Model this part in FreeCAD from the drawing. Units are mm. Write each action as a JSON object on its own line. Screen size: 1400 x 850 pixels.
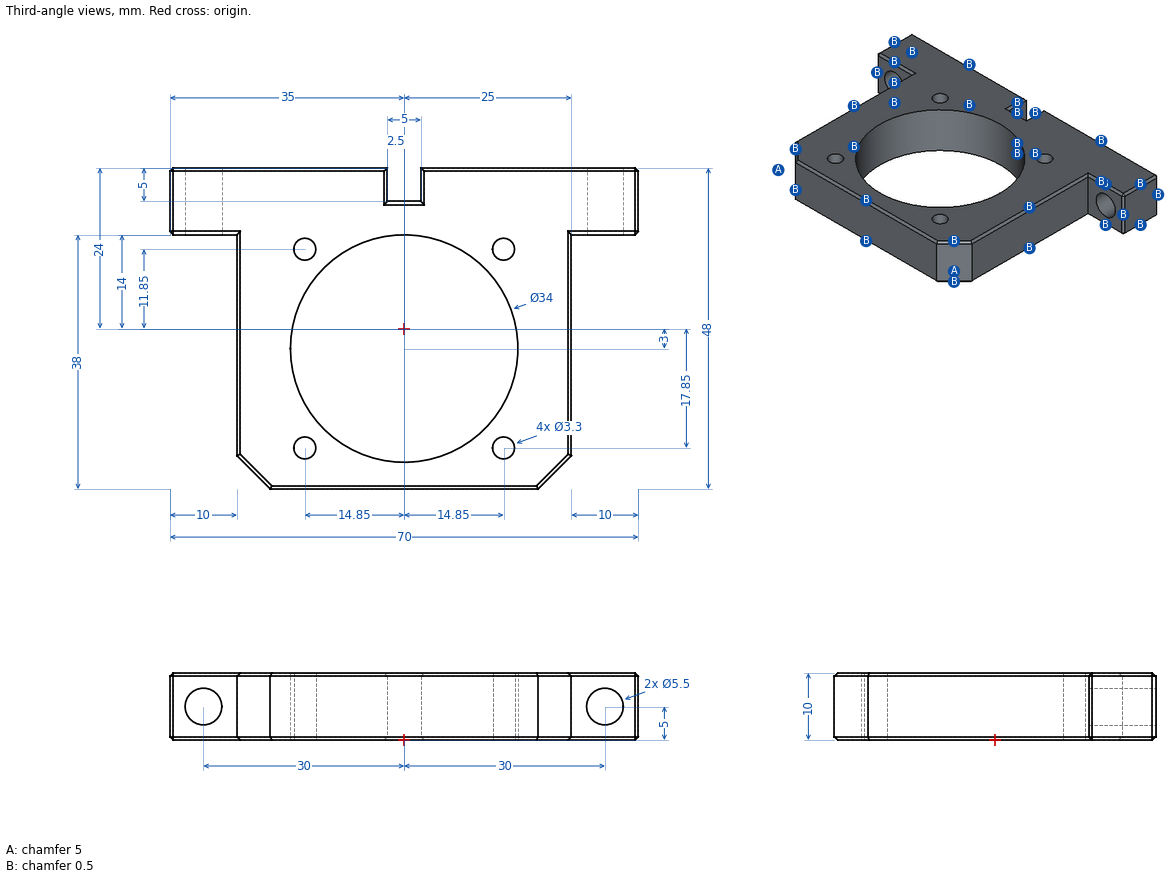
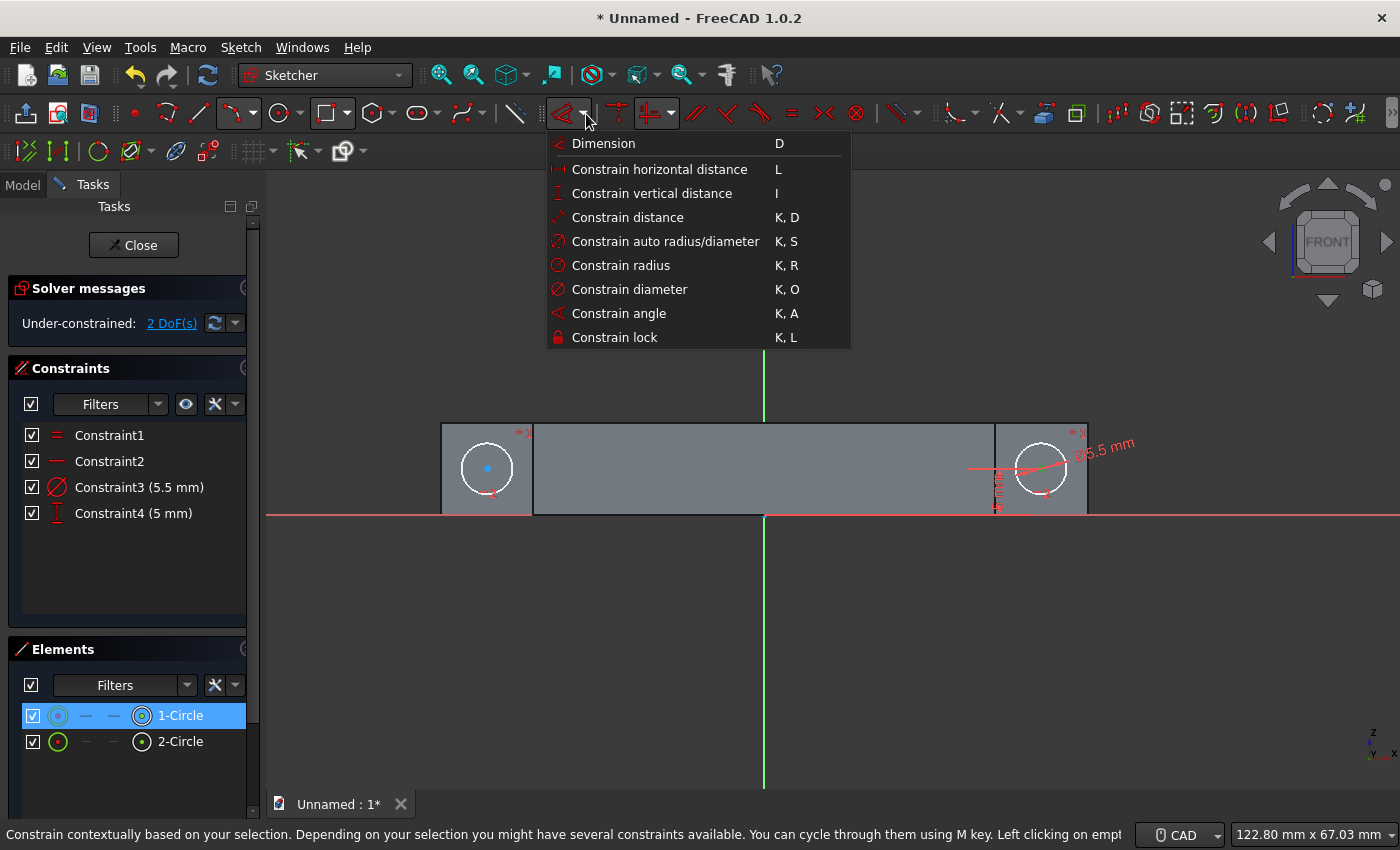
{"action": "left_click", "coordinate": [699, 169]}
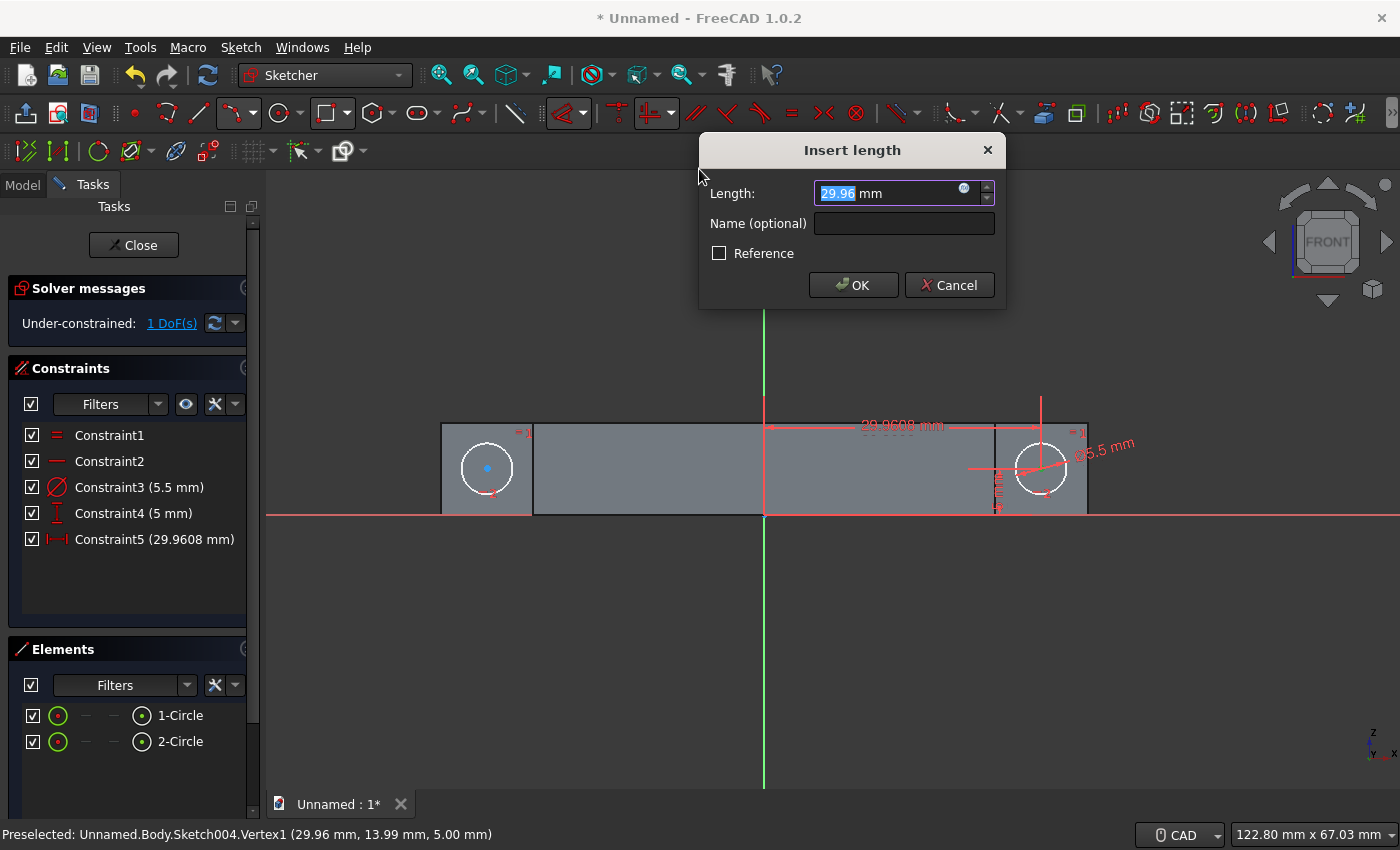
{"action": "type", "text": "30"}
{"action": "key", "text": "Return"}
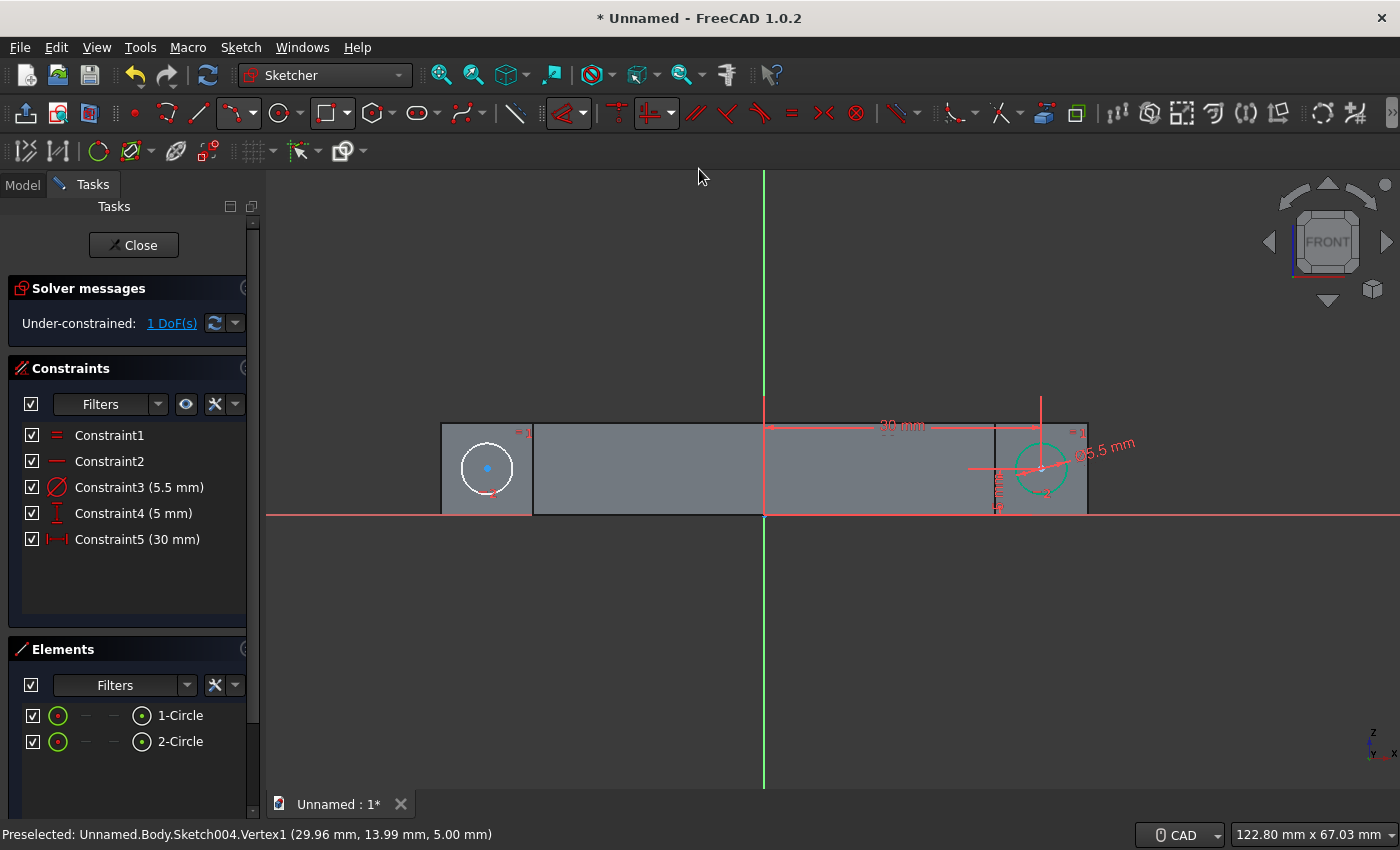
{"action": "left_click", "coordinate": [487, 469]}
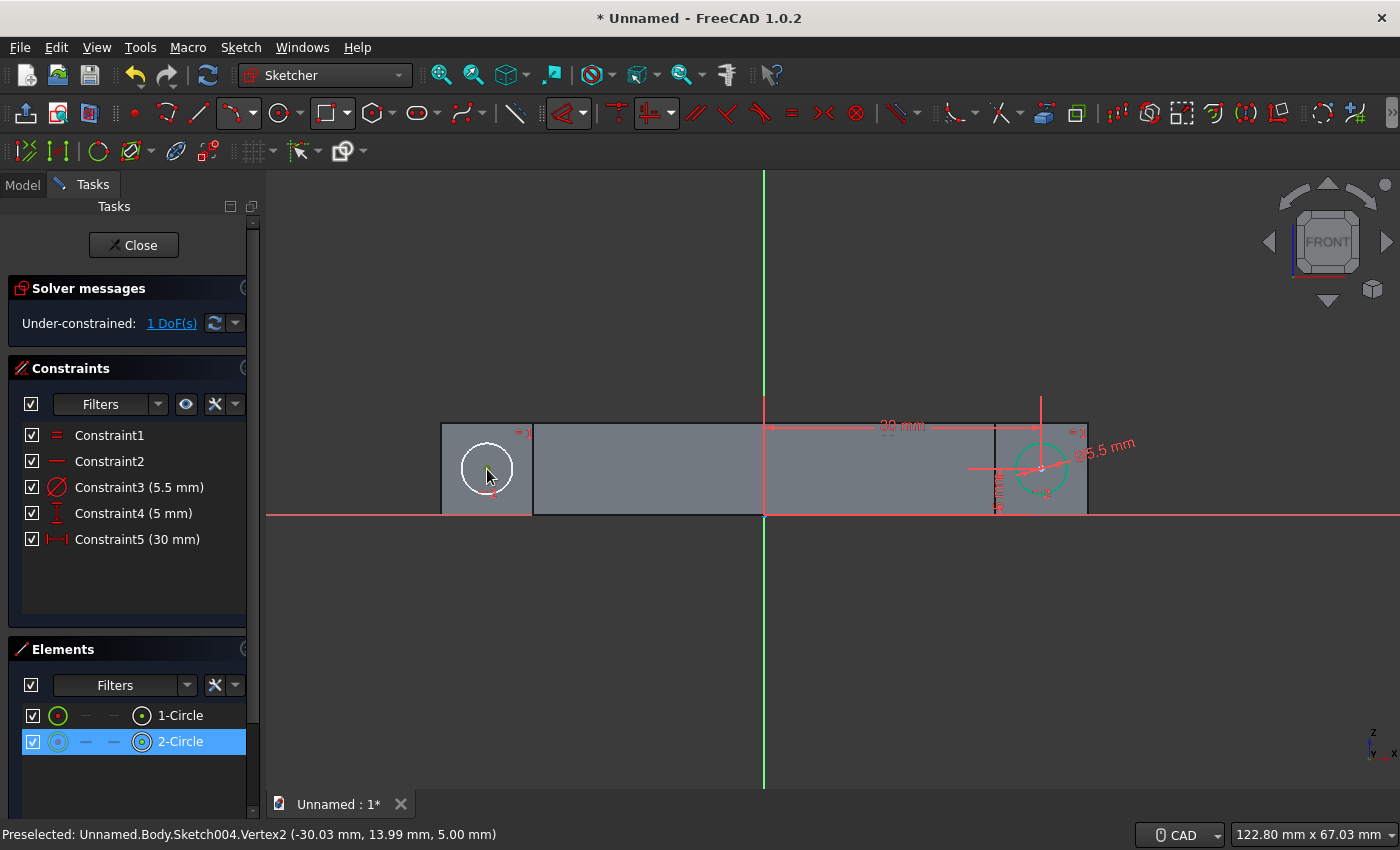
{"action": "key", "text": "l"}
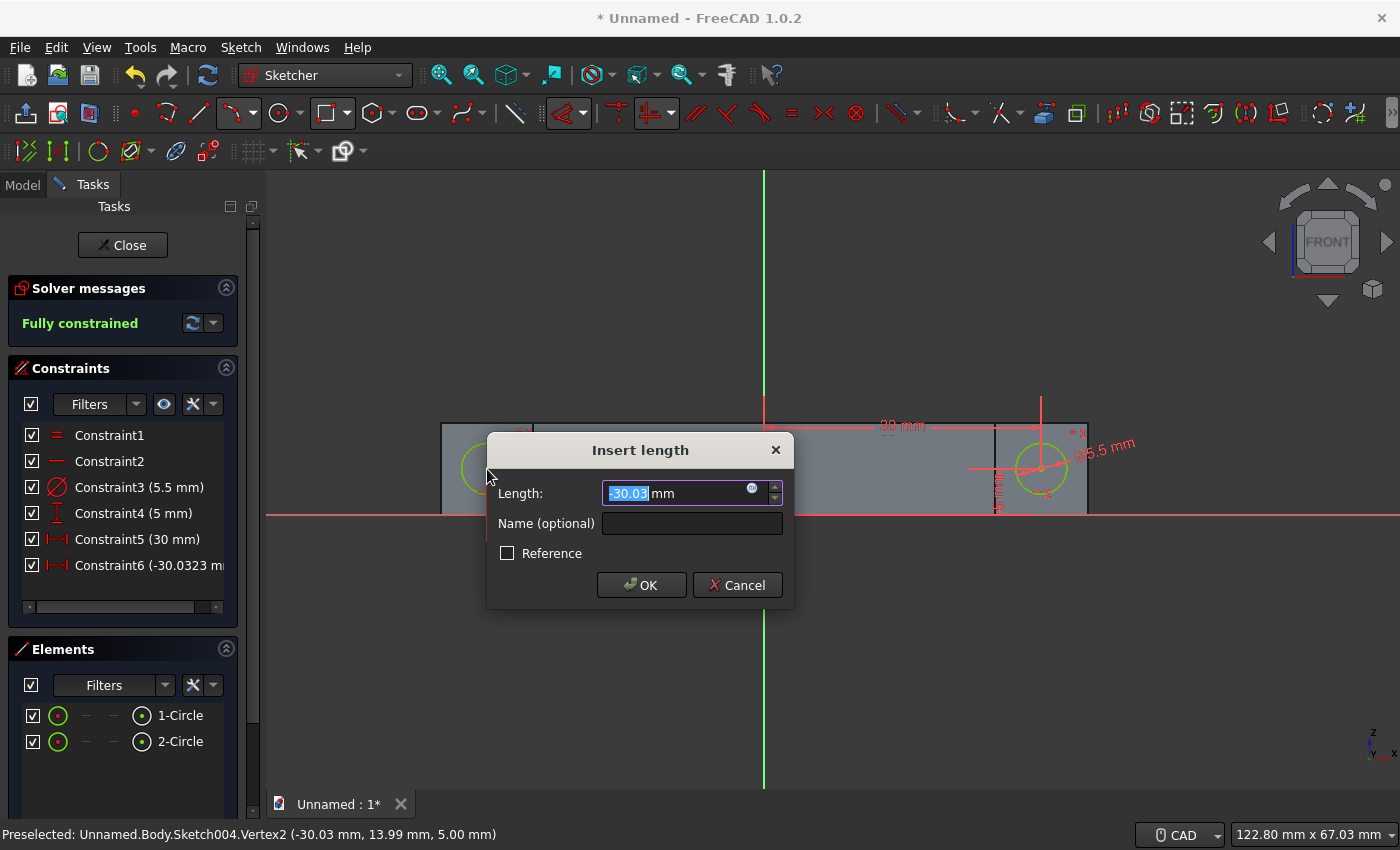
{"action": "type", "text": "-30"}
{"action": "key", "text": "Return"}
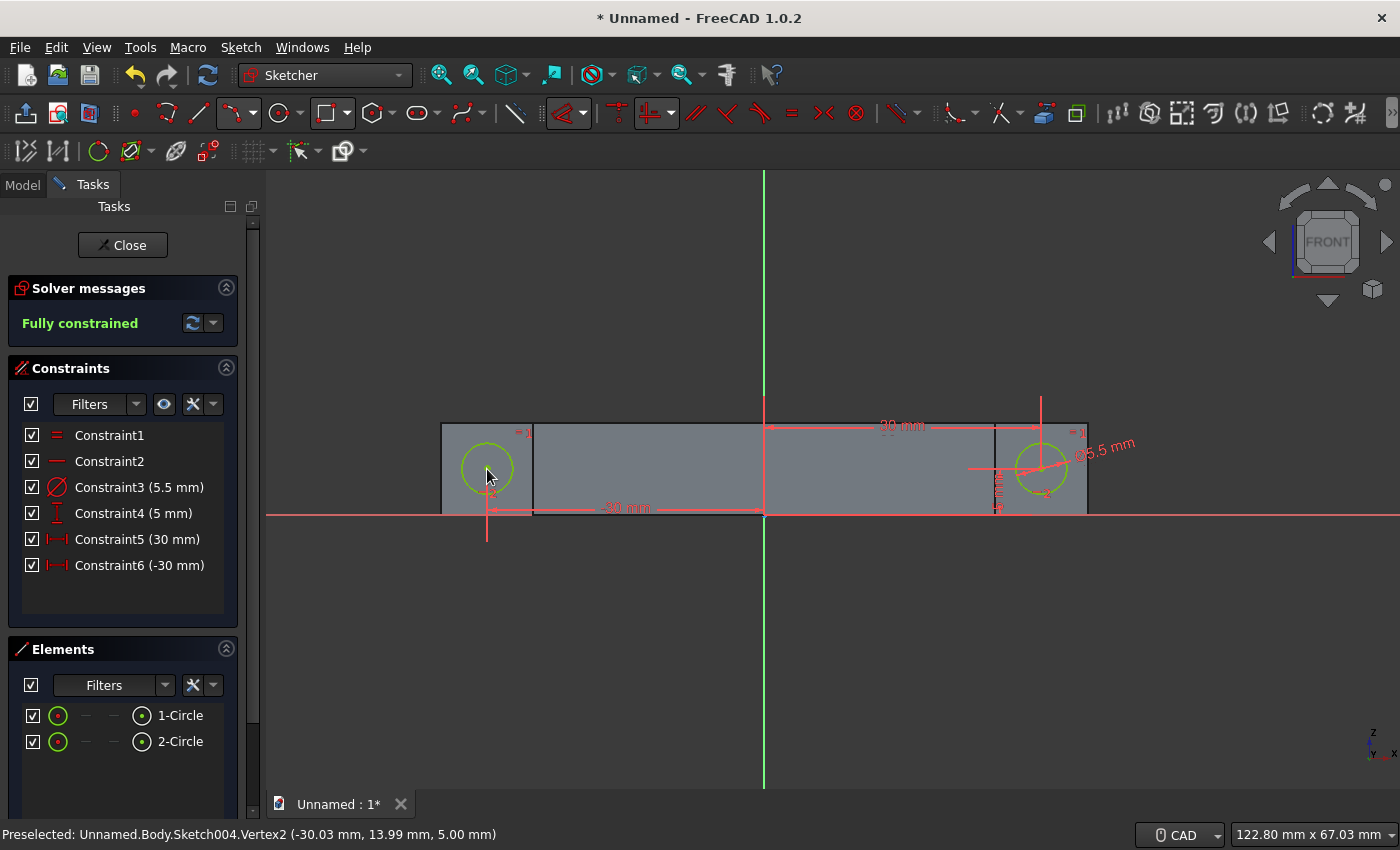
{"action": "left_click", "coordinate": [123, 245]}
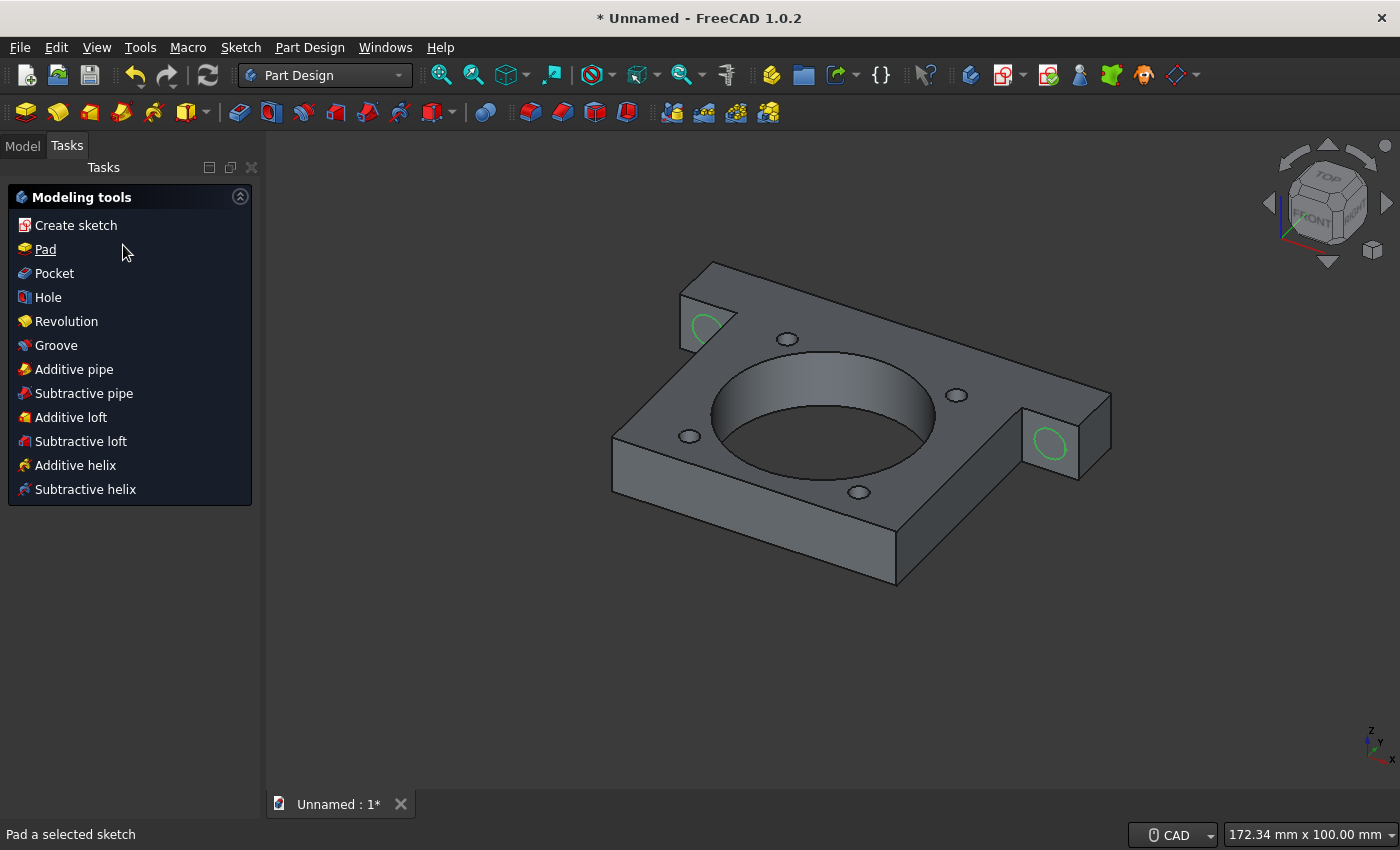
{"action": "left_click", "coordinate": [240, 112]}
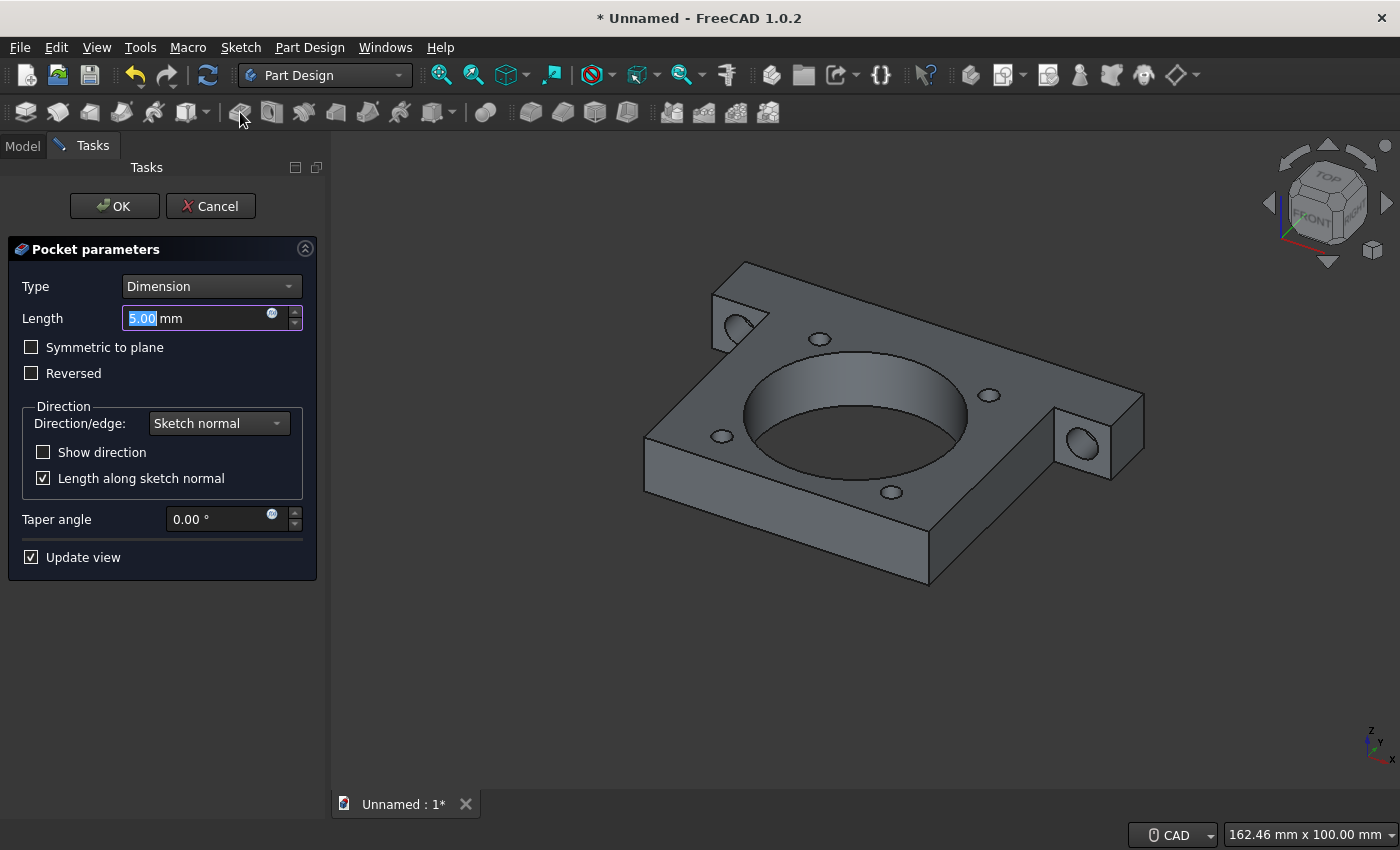
{"action": "left_click", "coordinate": [212, 286]}